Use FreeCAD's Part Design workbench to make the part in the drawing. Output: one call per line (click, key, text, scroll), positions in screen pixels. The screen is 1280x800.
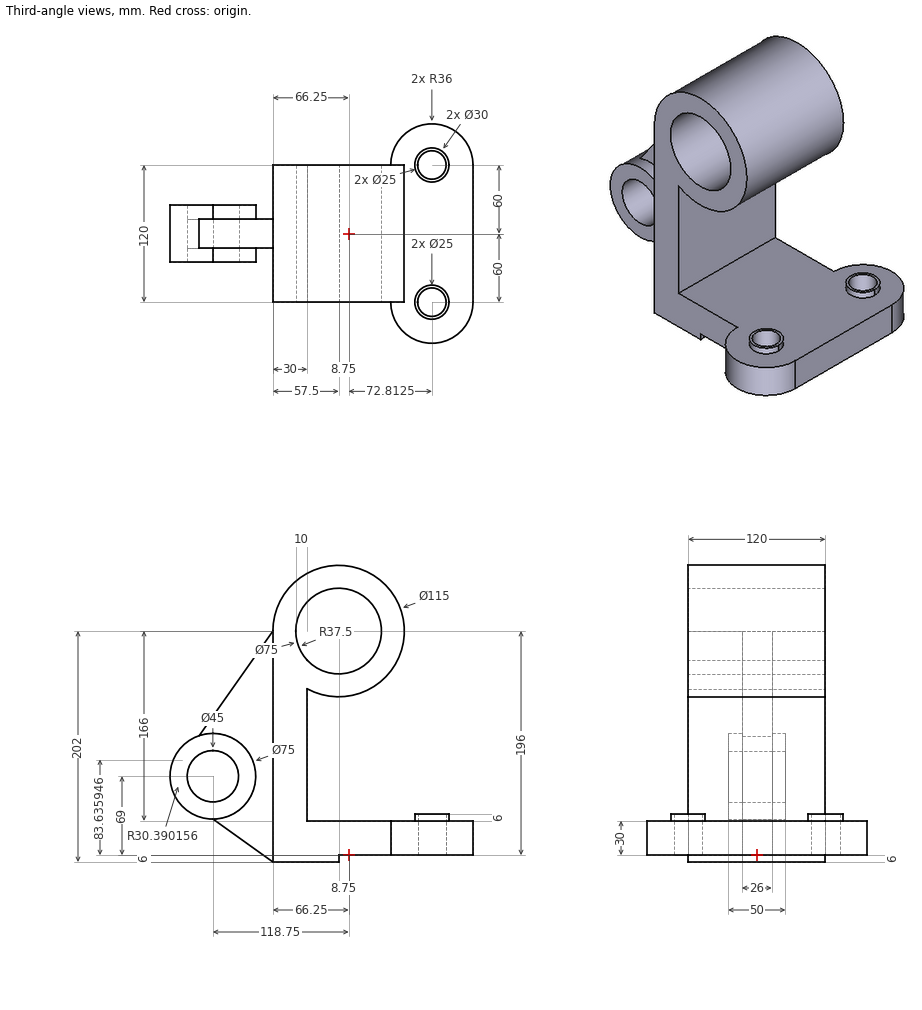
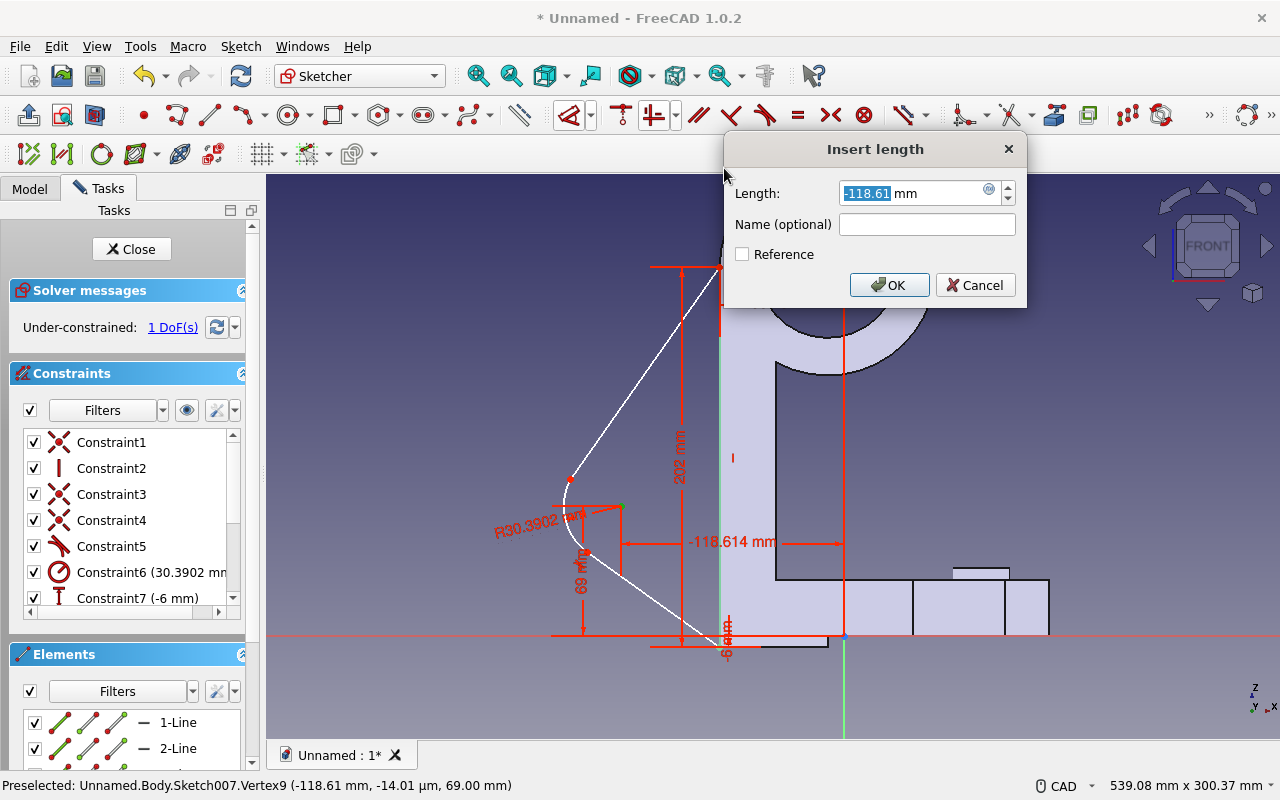
text(-118.75)
key(Return)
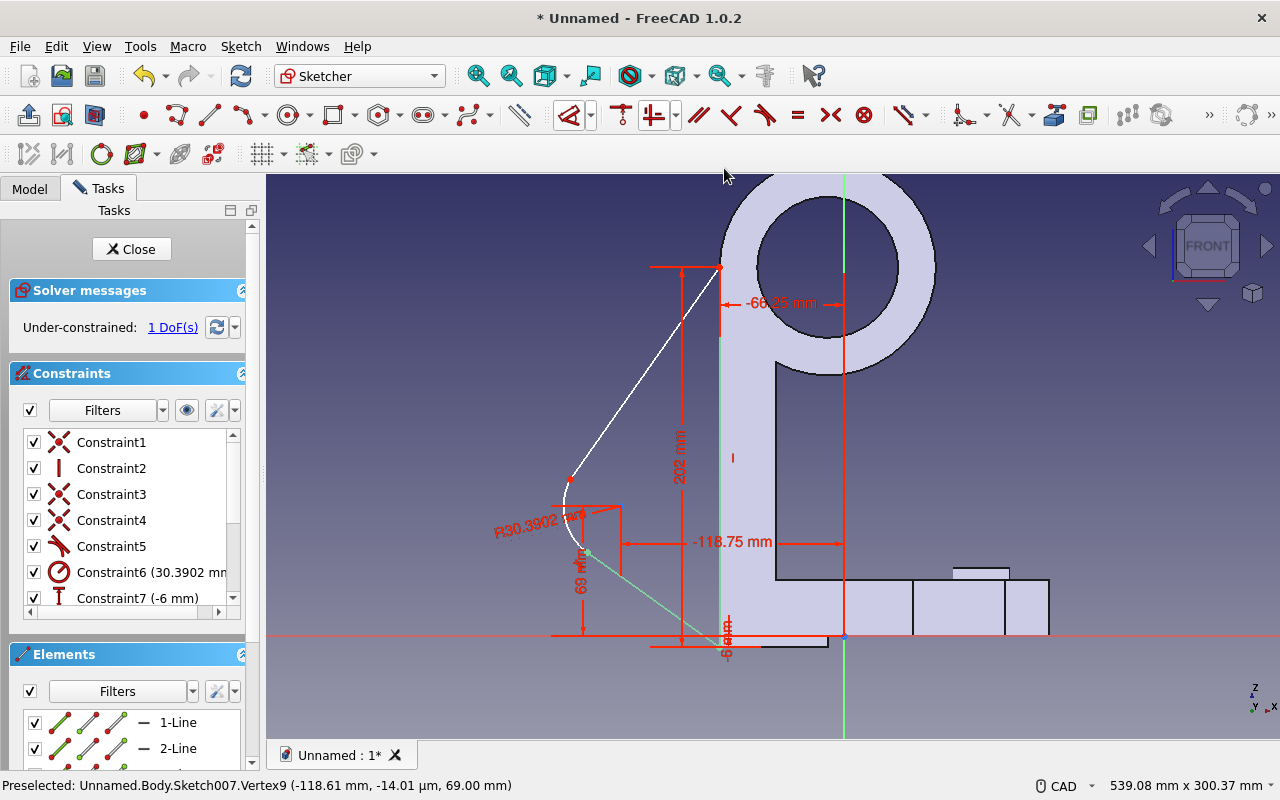
click(570, 480)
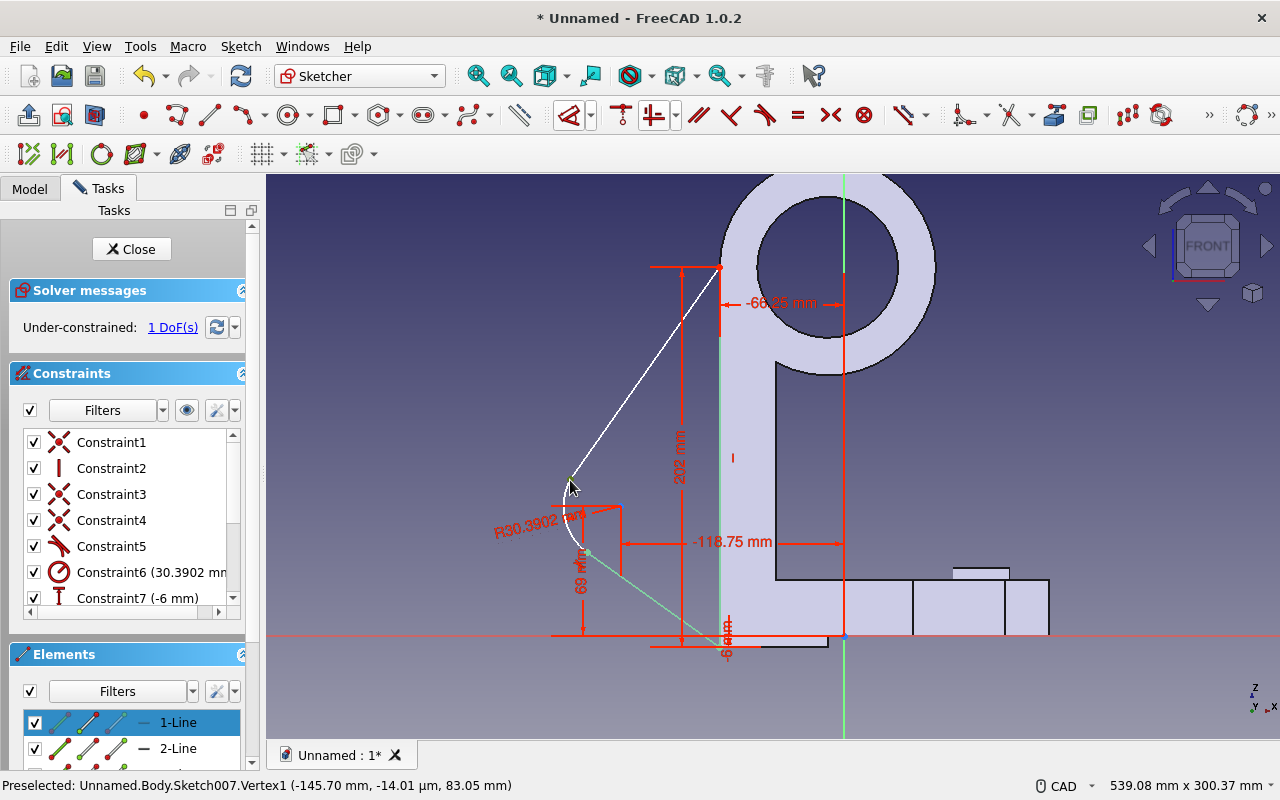
key(i)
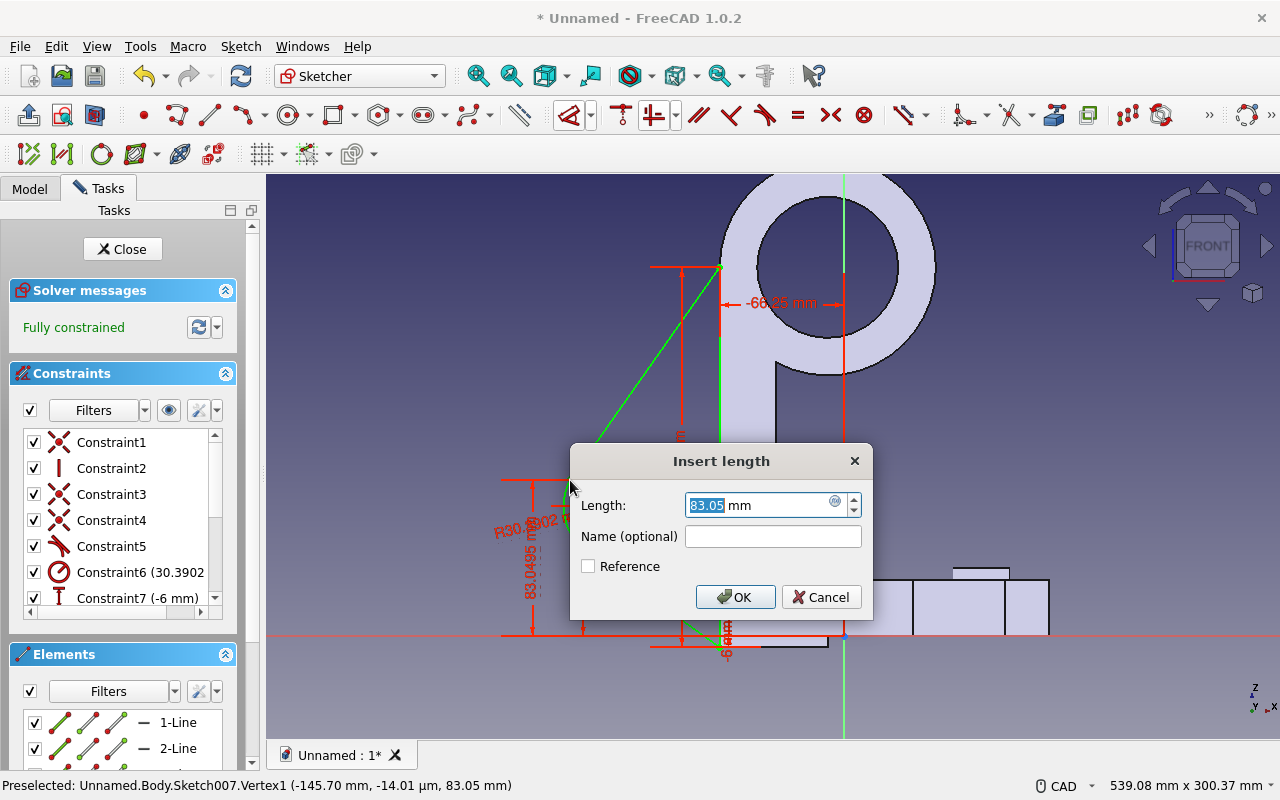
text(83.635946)
key(Return)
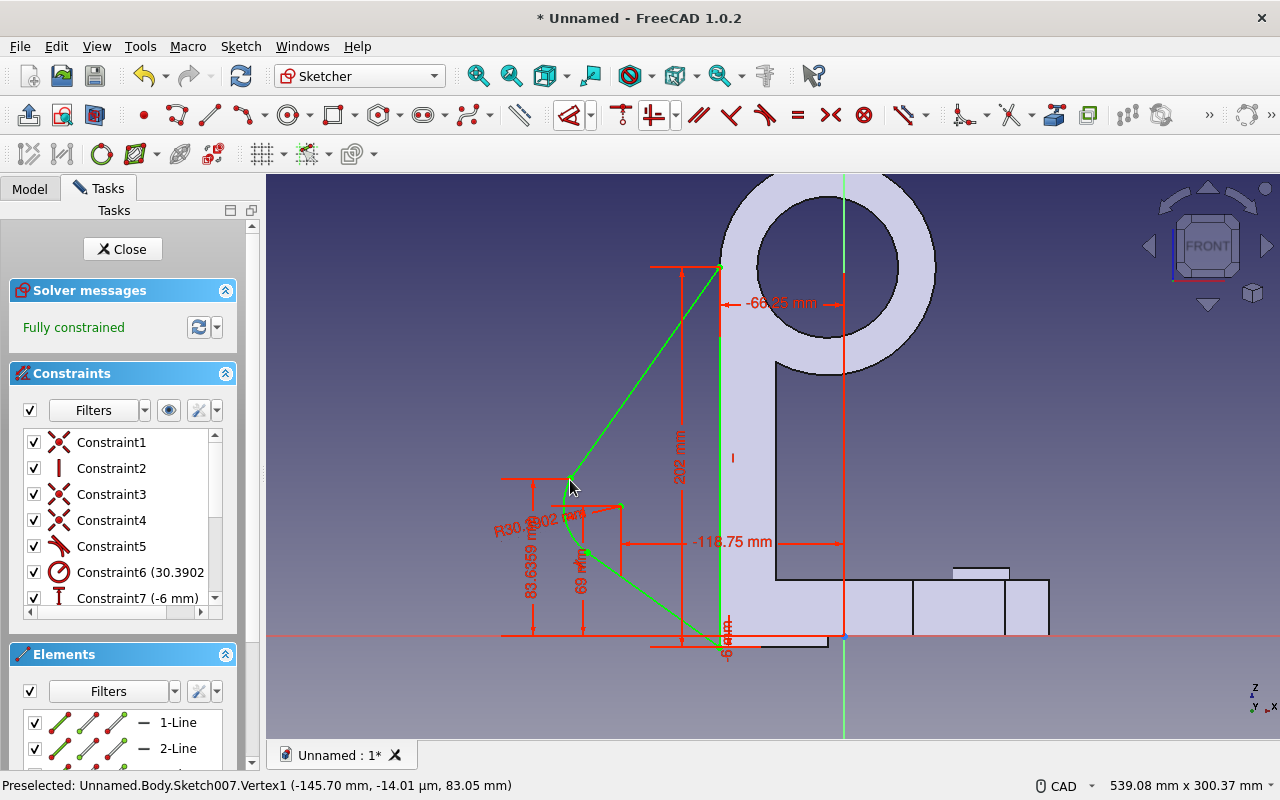
click(123, 249)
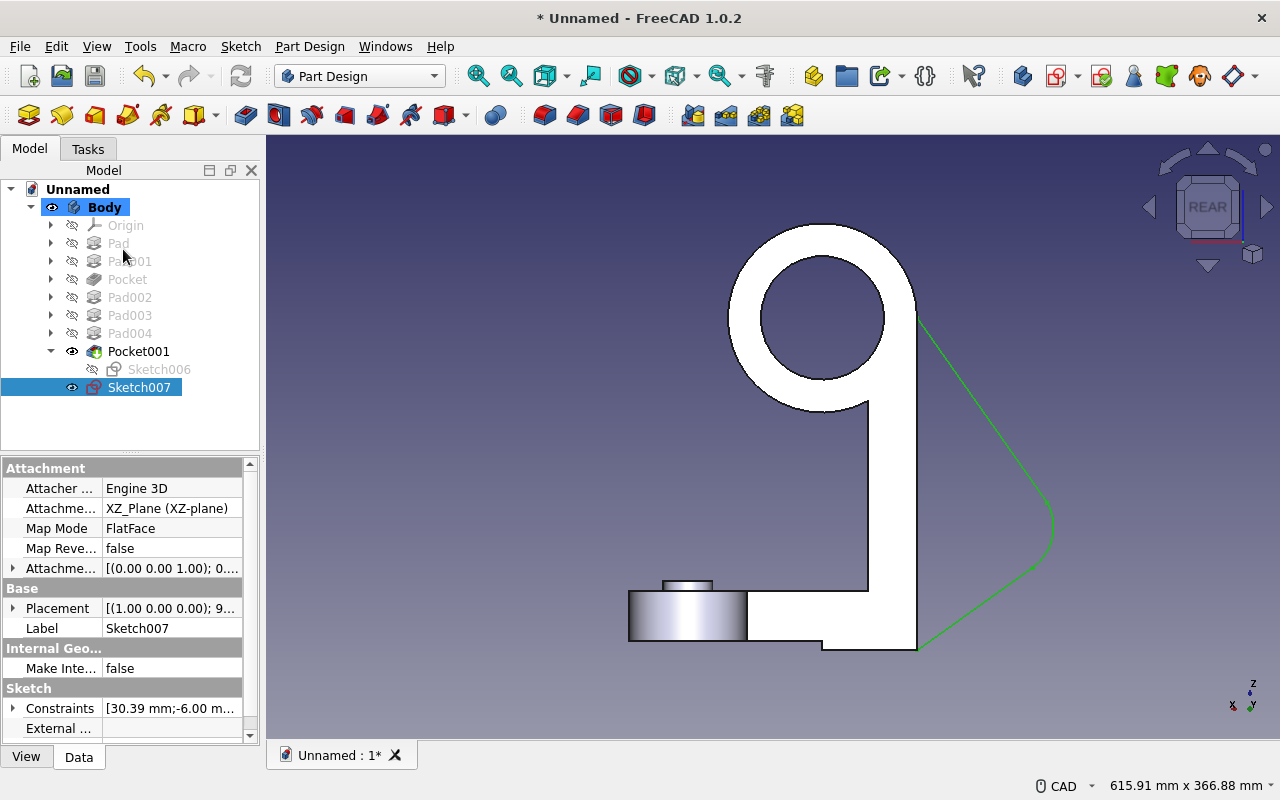
click(29, 116)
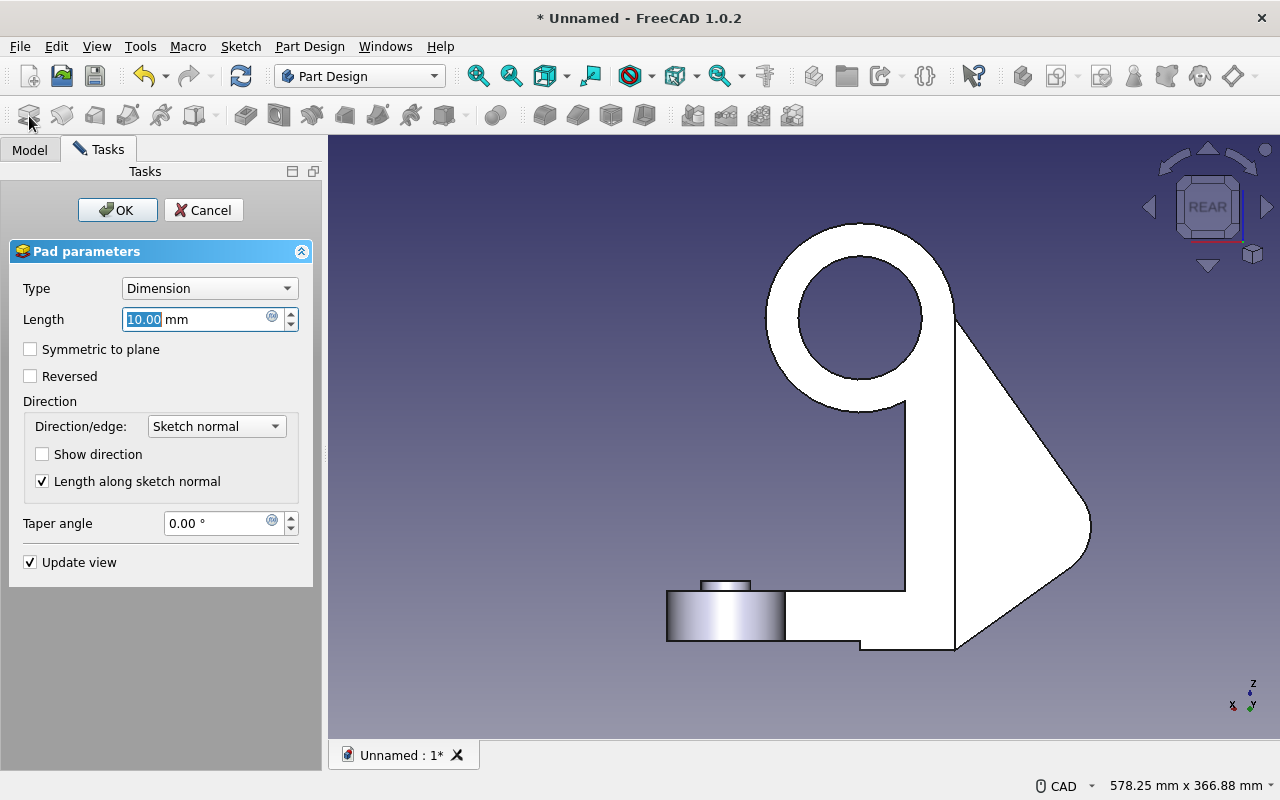
text(26)
key(Tab)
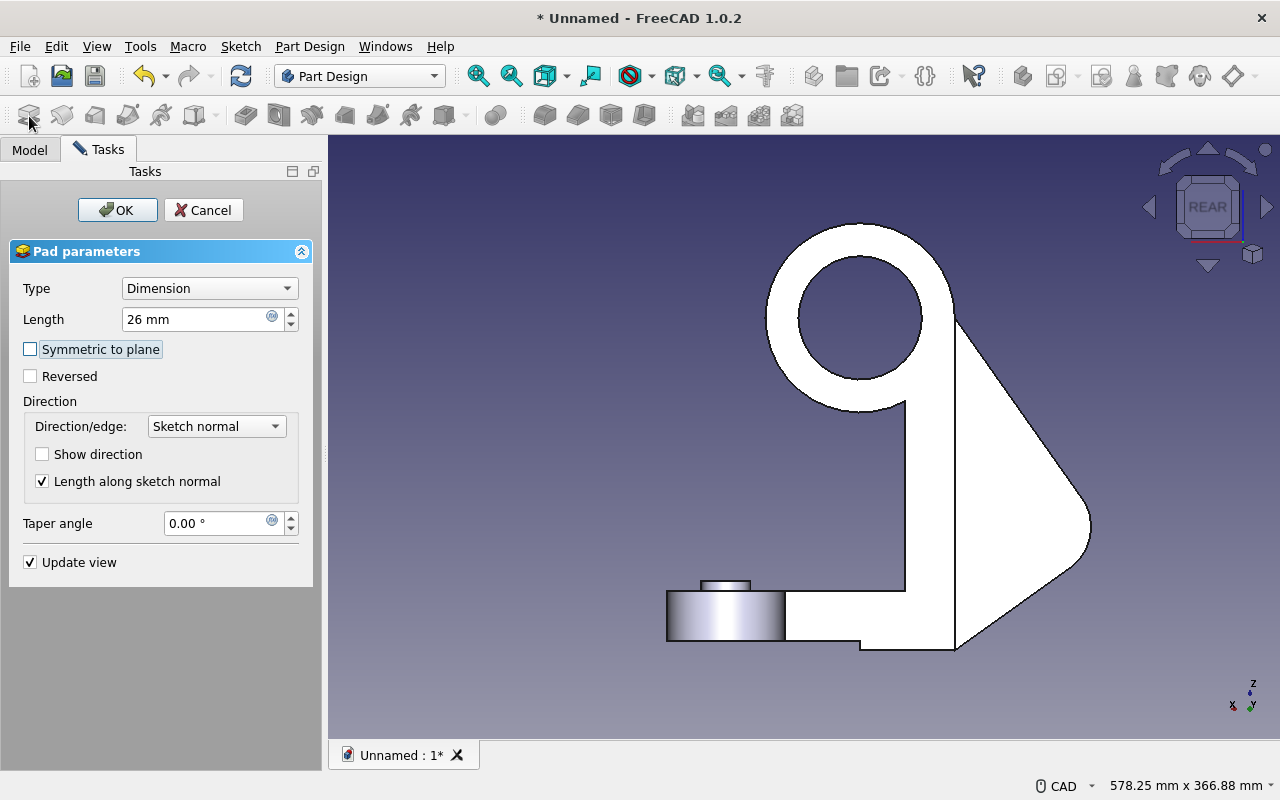
click(31, 349)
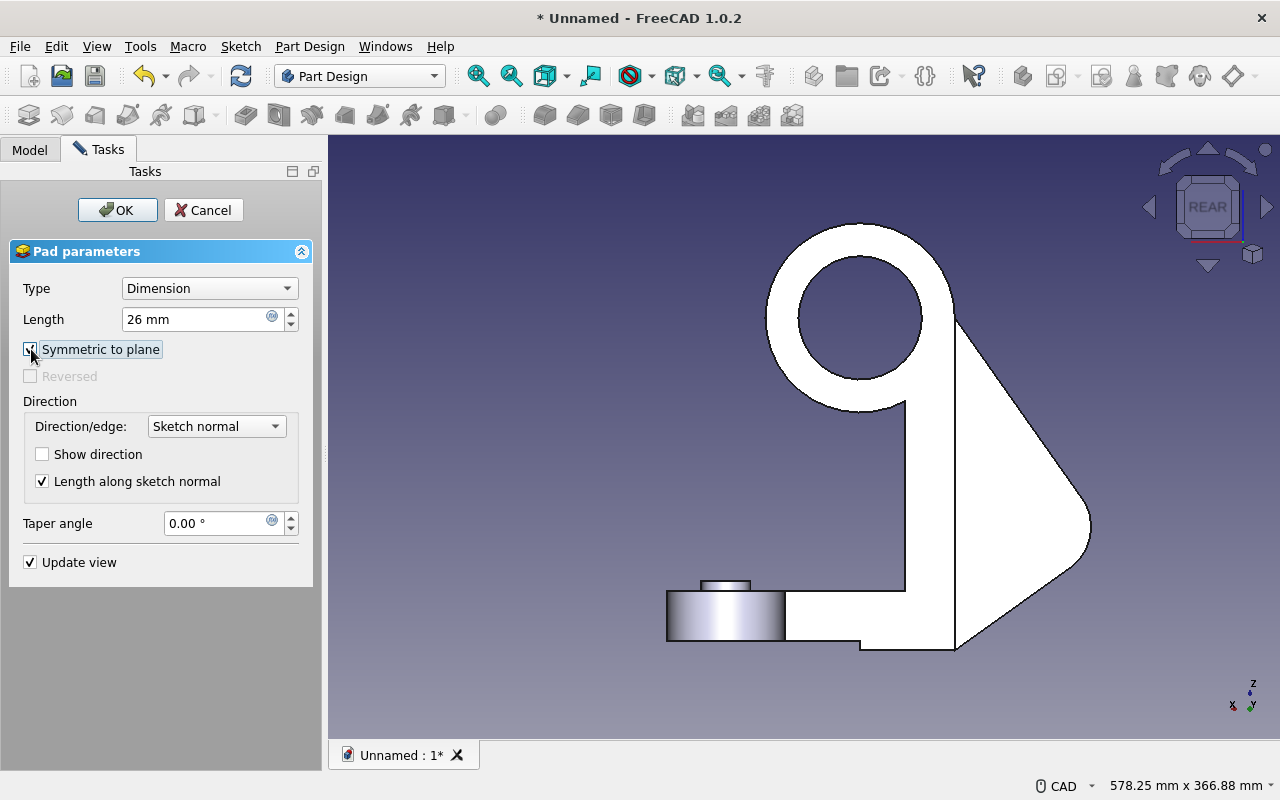
click(118, 210)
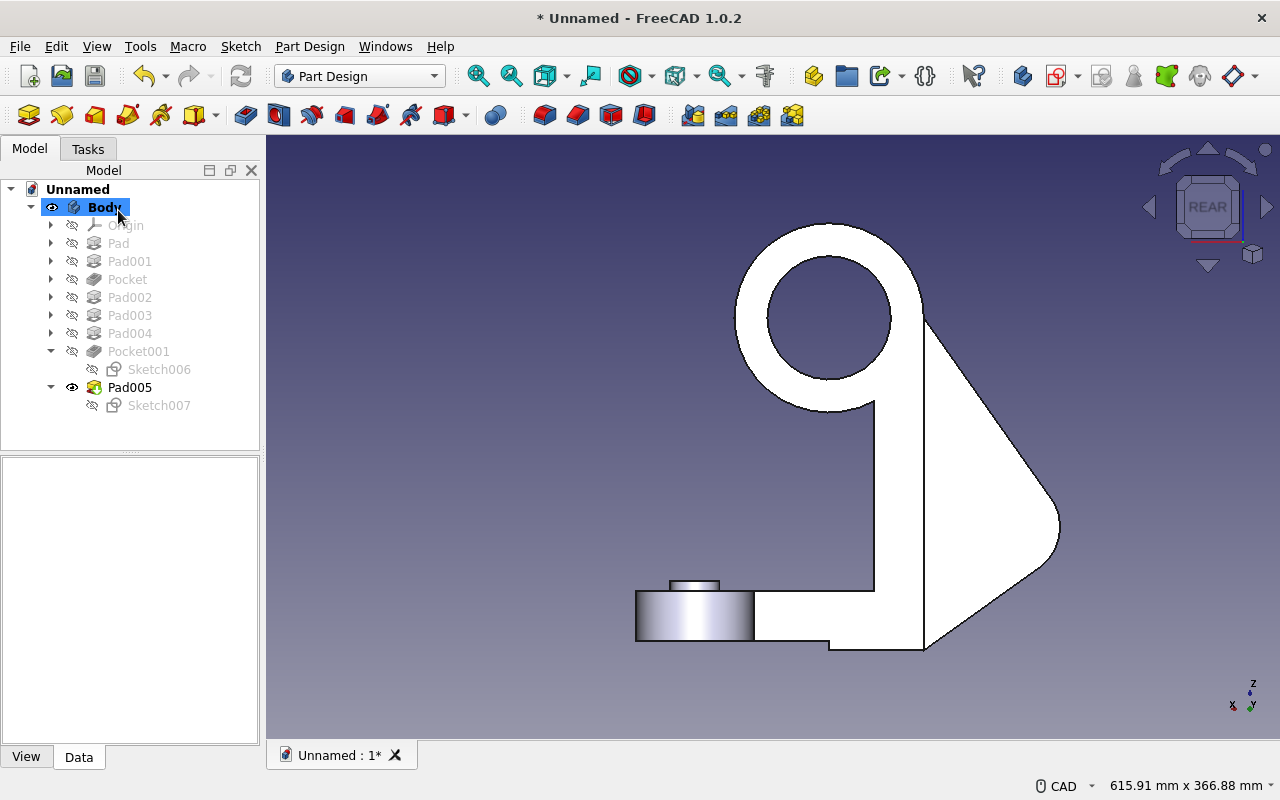
click(1056, 76)